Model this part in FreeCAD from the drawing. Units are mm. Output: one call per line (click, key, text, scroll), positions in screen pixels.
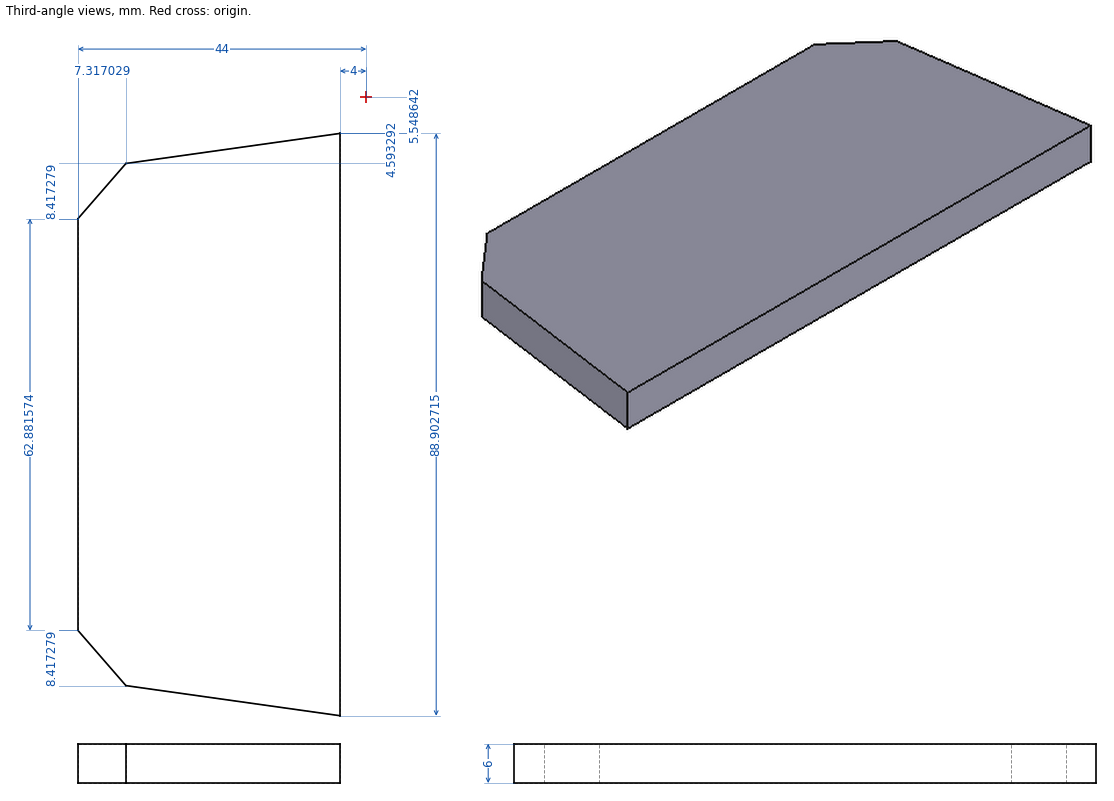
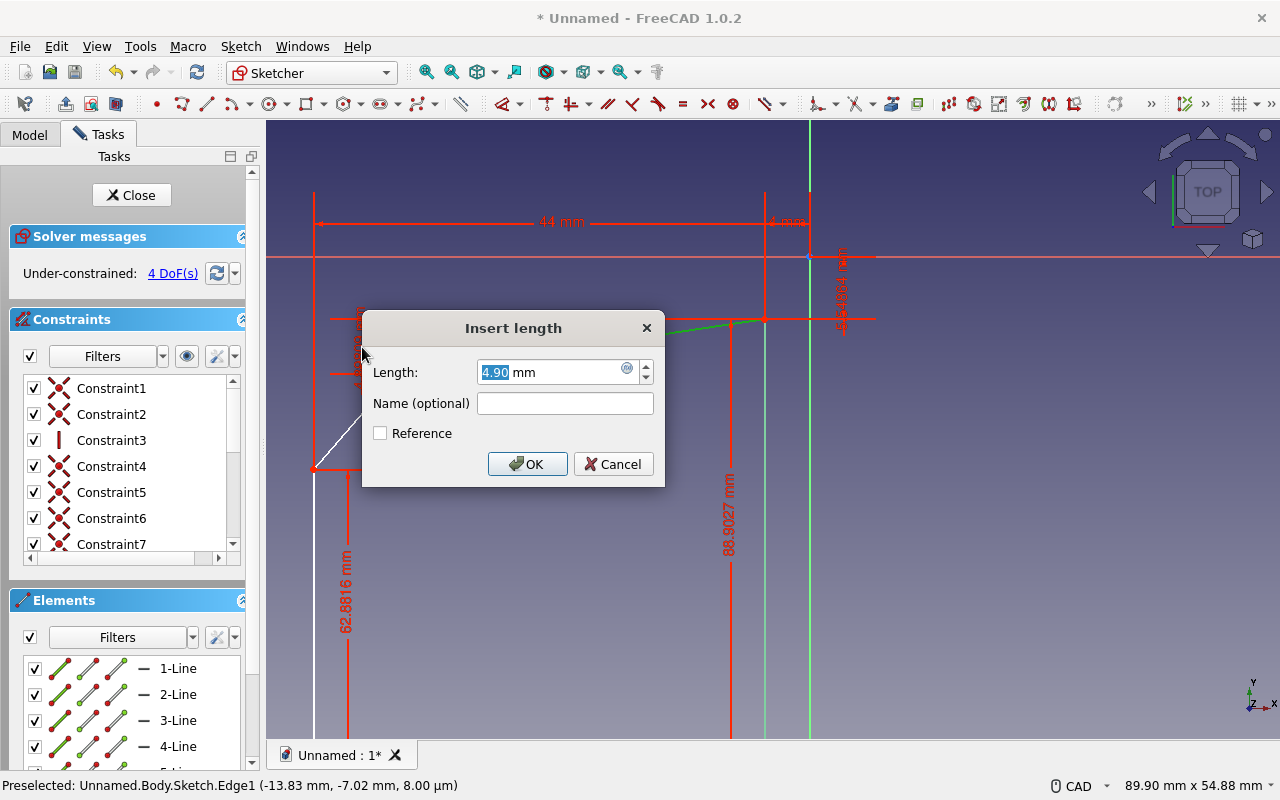
text(4.593292)
key(Return)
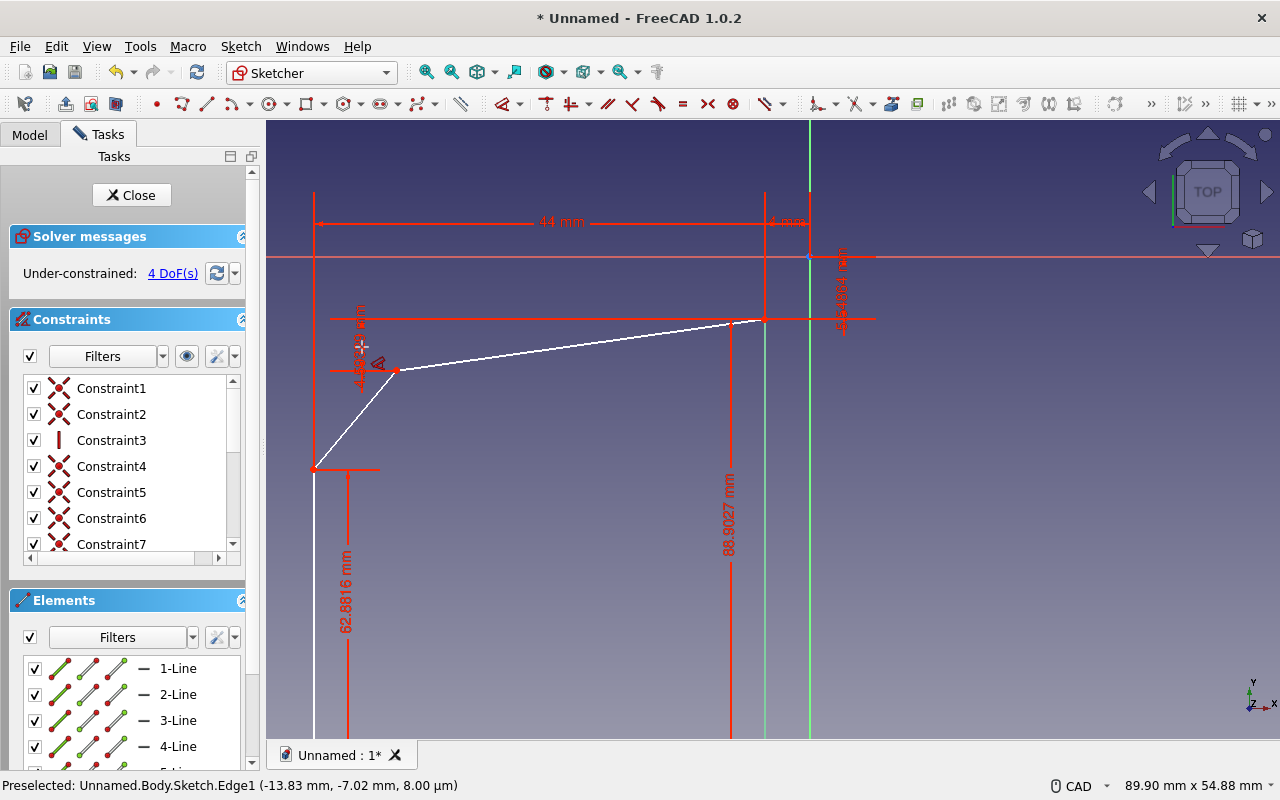
click(371, 401)
click(355, 504)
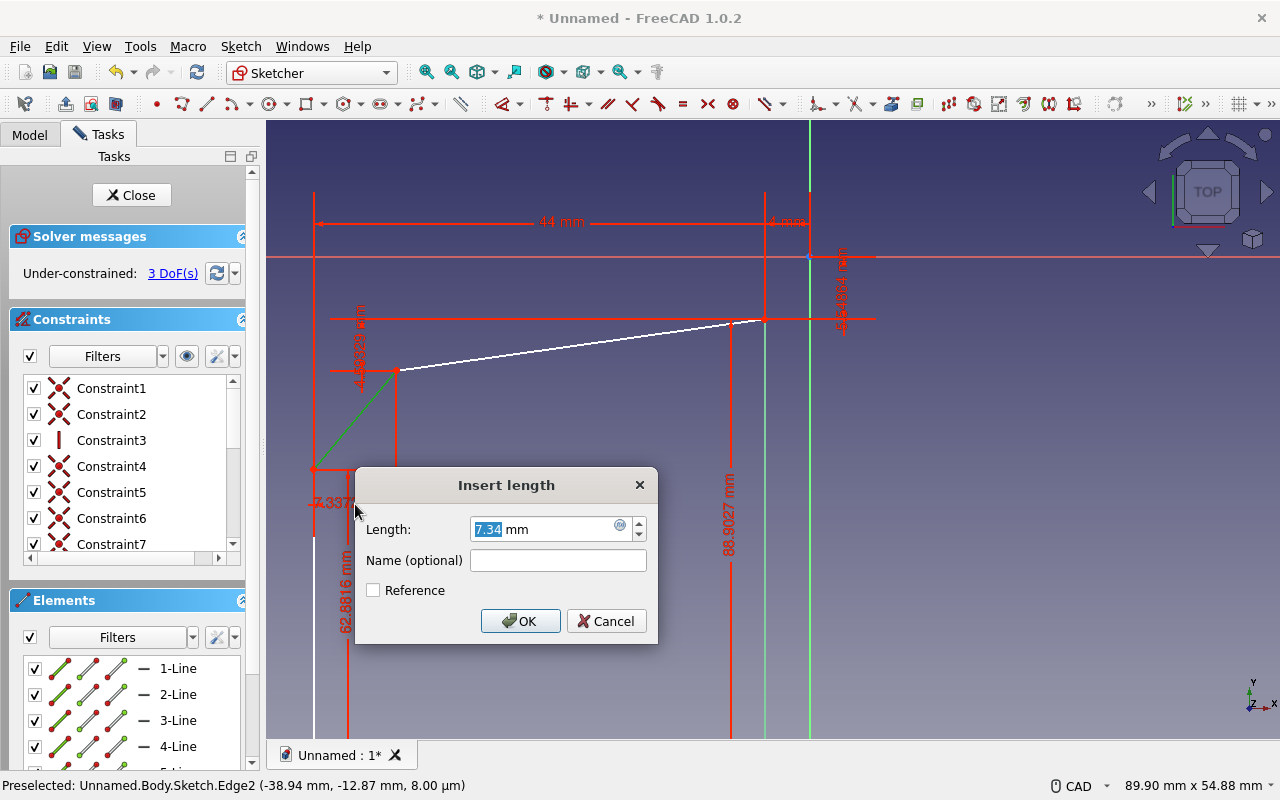
text(7.317029)
key(Return)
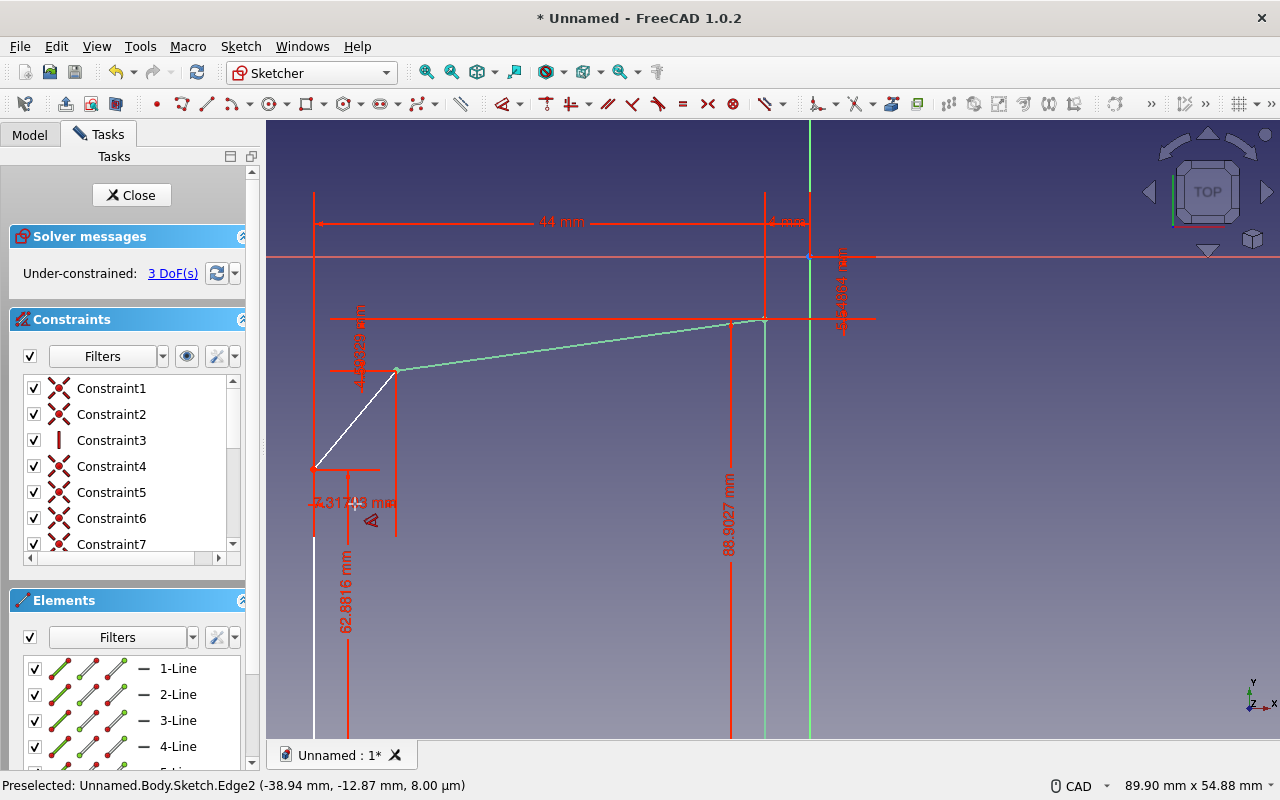
click(371, 401)
click(430, 420)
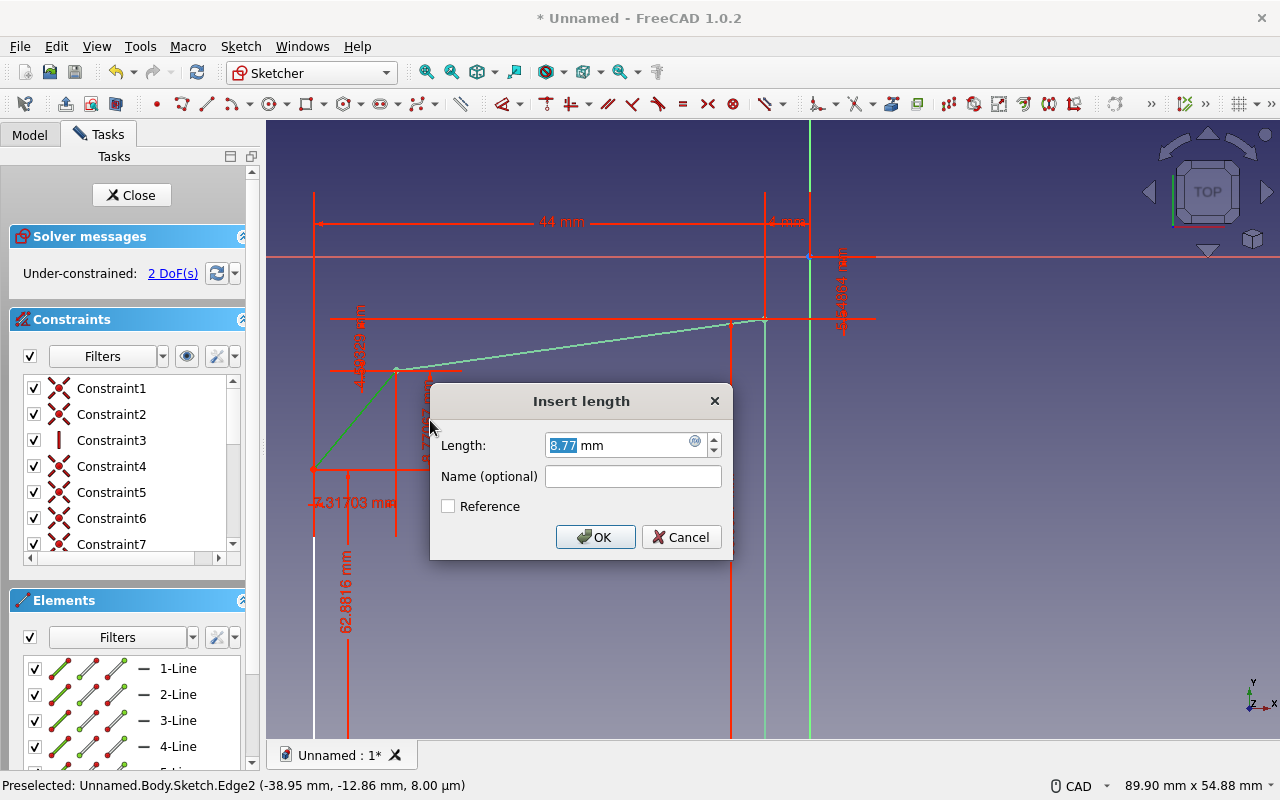
text(8.417279)
key(Return)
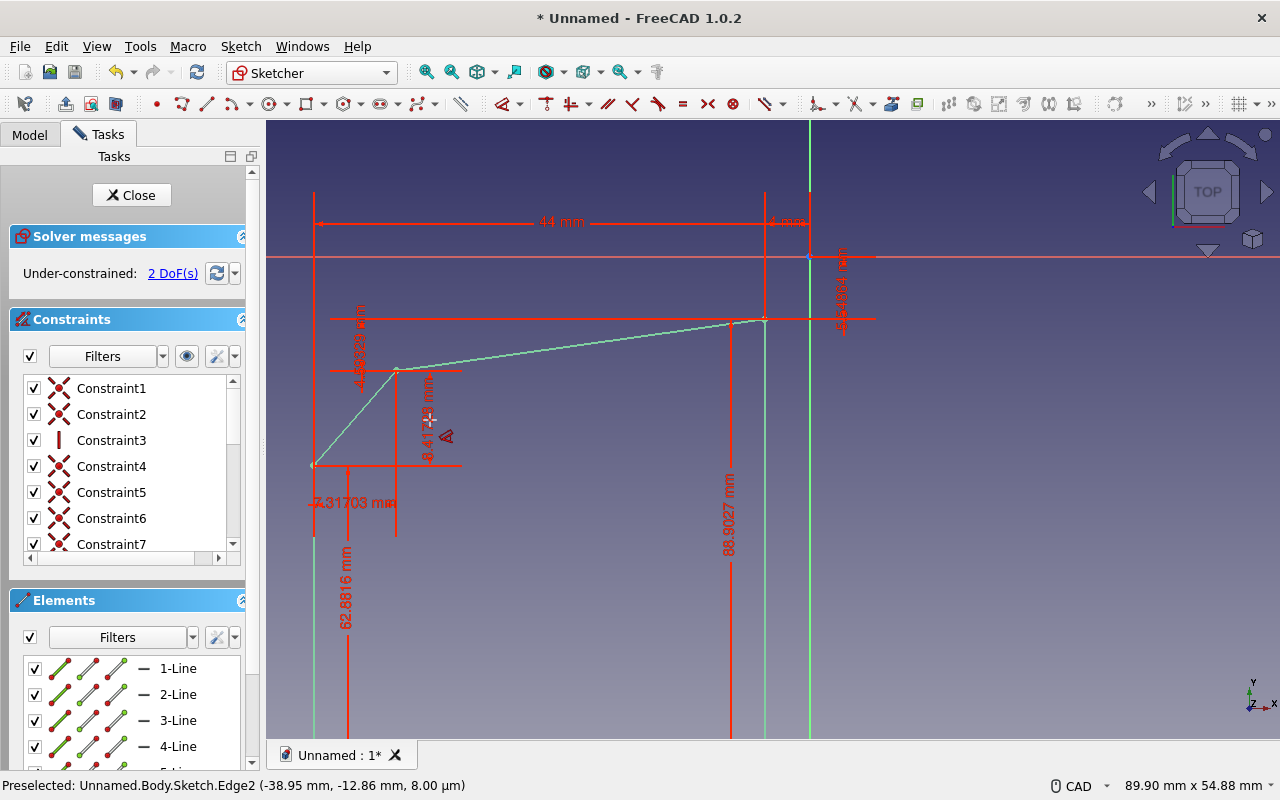
scroll(788, 220, down, 5)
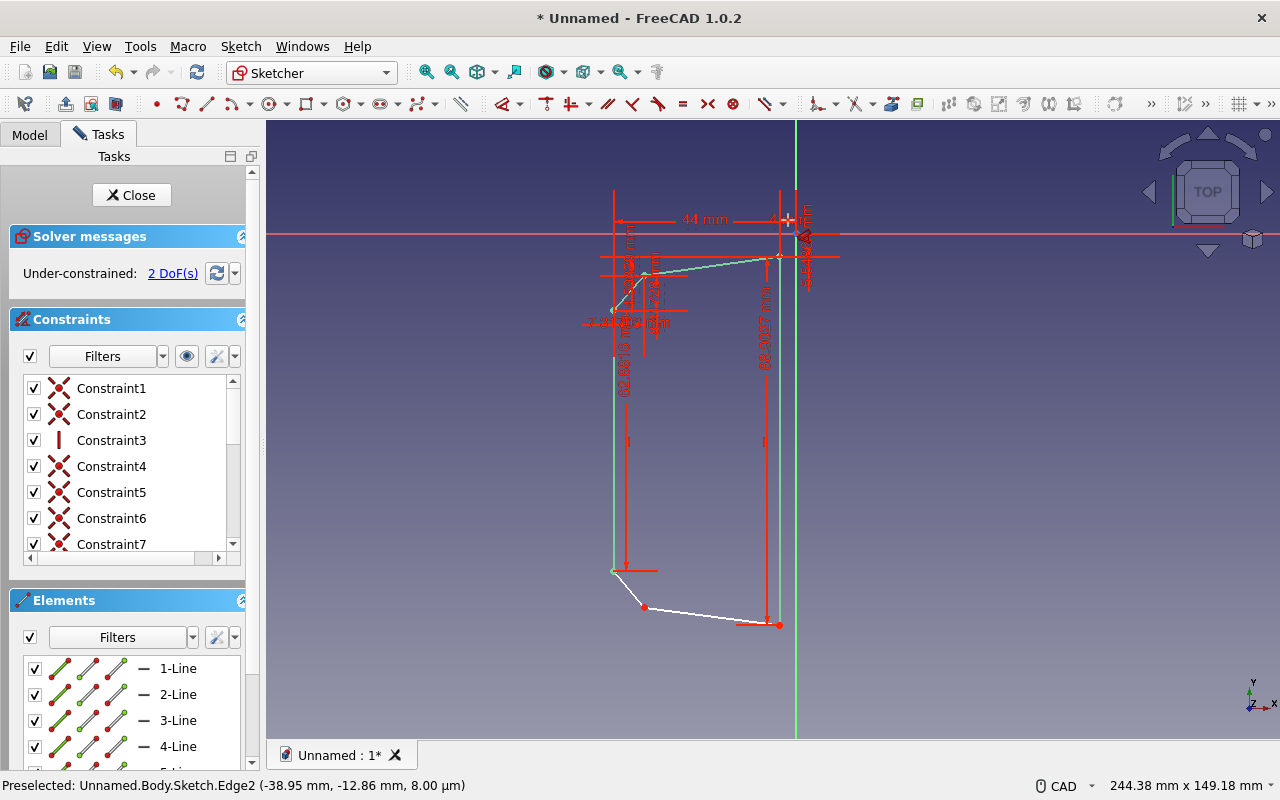
scroll(623, 582, up, 2)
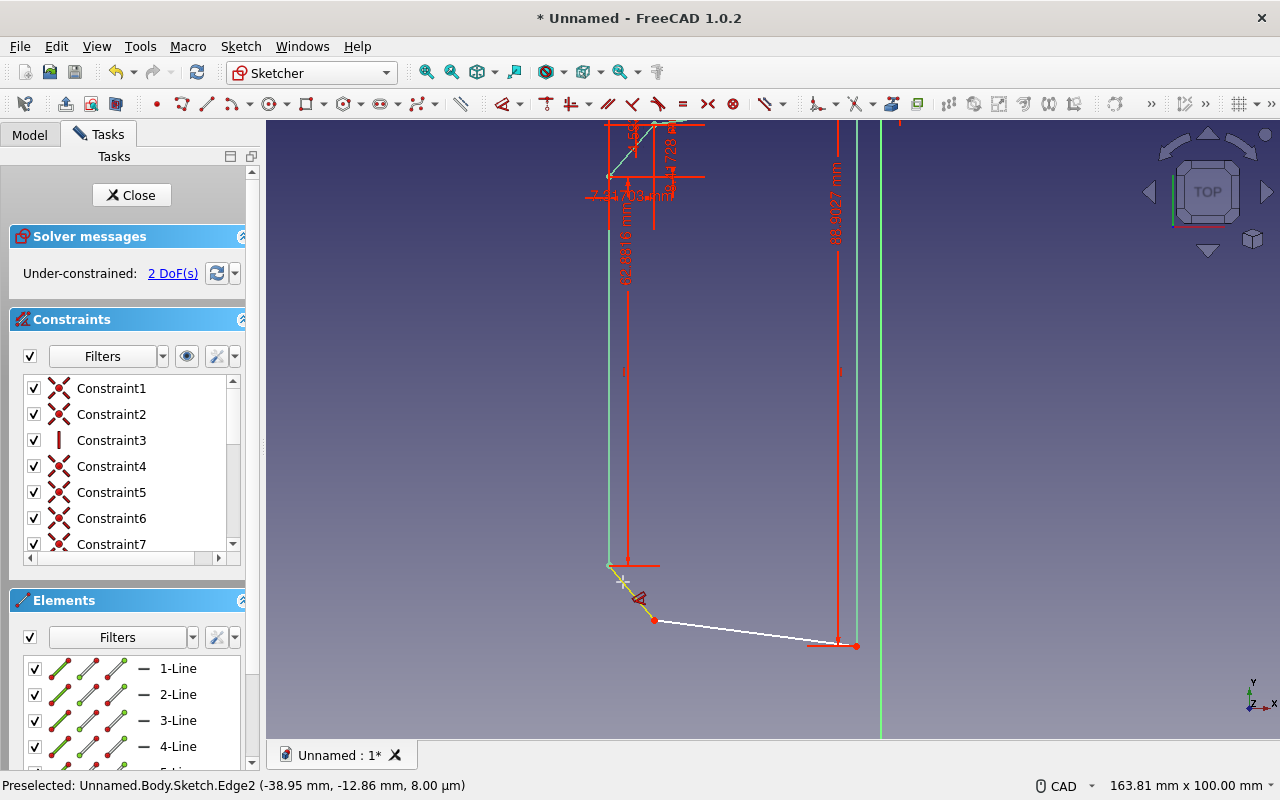
click(623, 582)
click(632, 654)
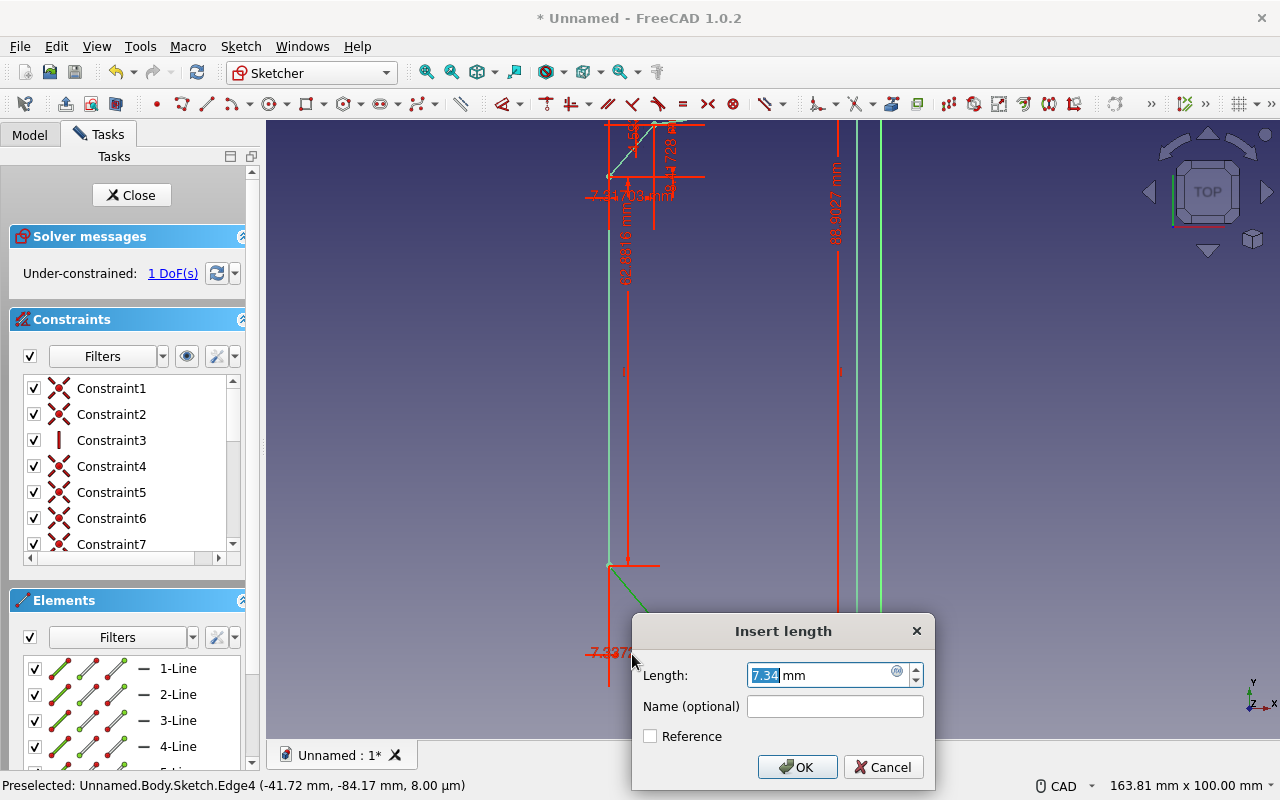
text(7.317029)
key(Return)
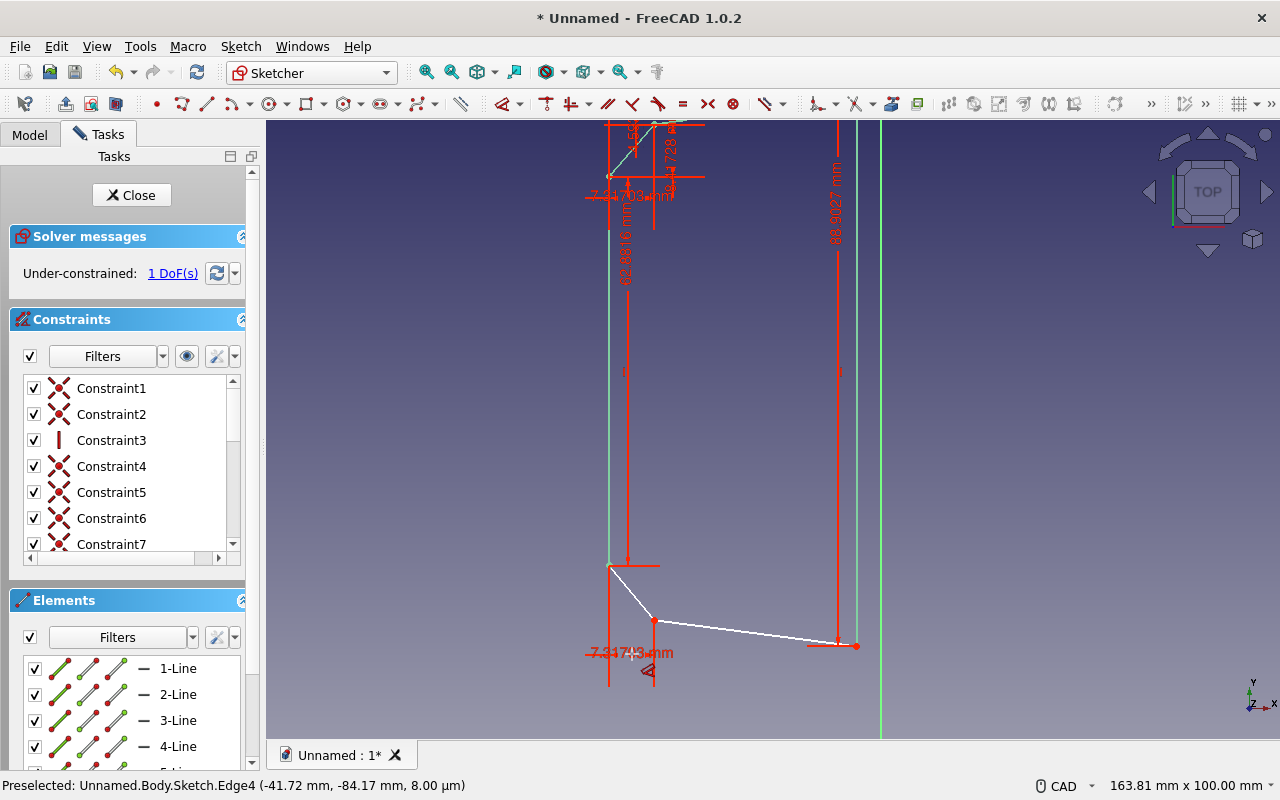
click(623, 582)
click(575, 593)